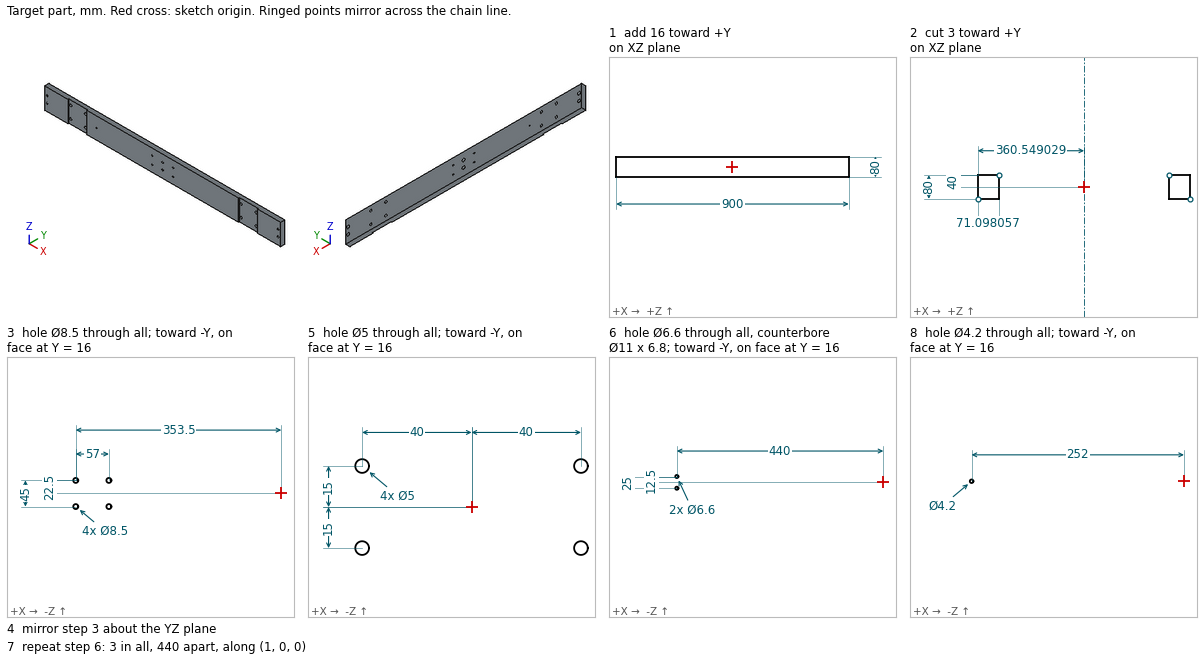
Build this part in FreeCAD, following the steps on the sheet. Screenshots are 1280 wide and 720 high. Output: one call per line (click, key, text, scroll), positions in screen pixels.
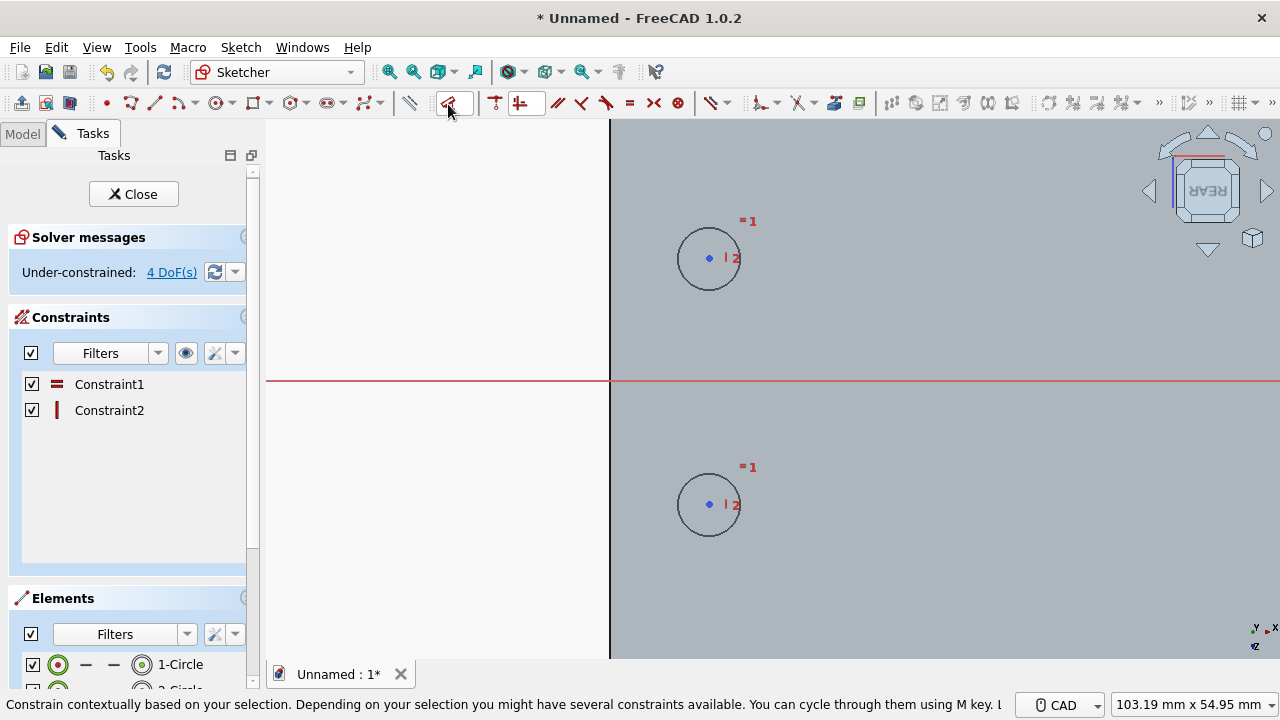
click(731, 237)
click(754, 214)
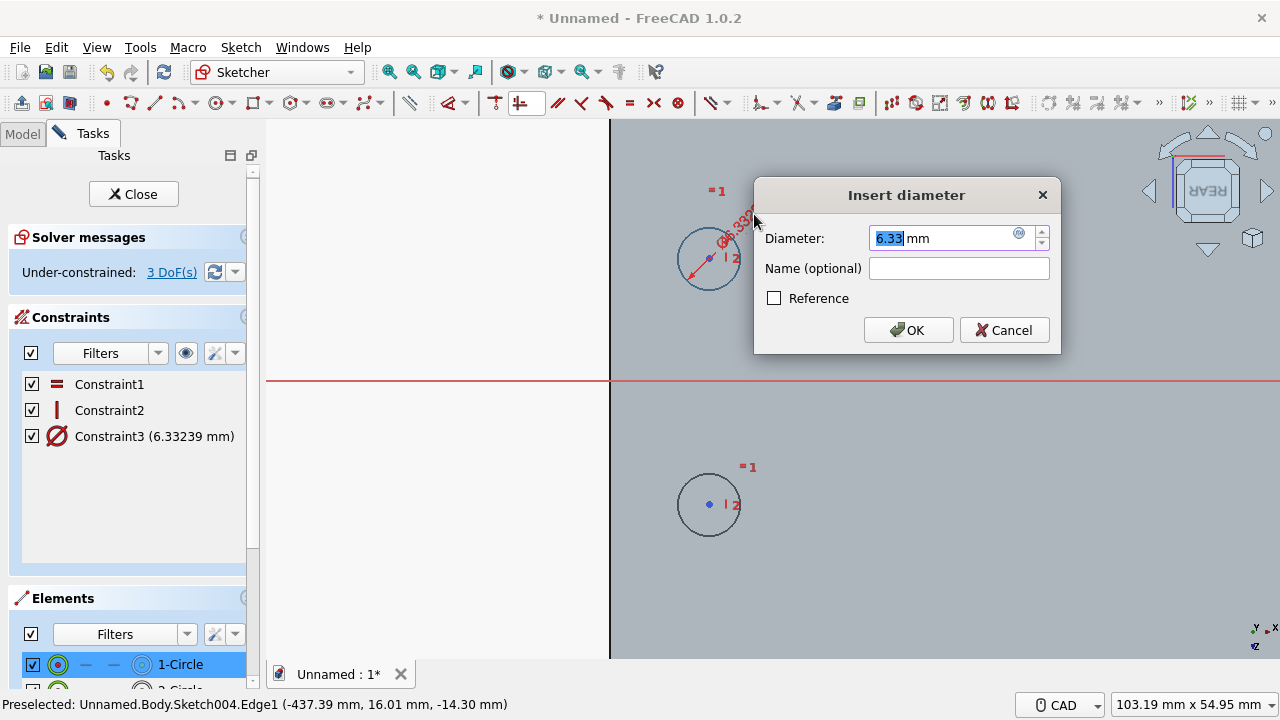
text(6.6)
key(Return)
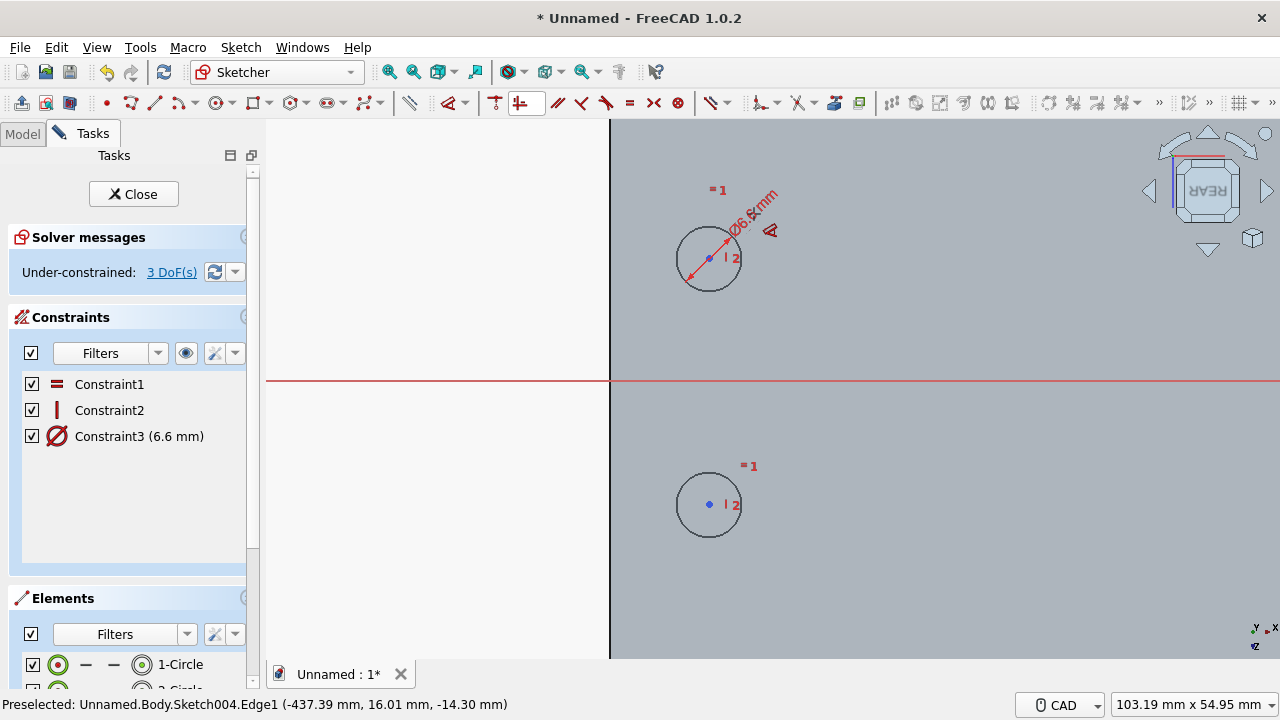
click(709, 259)
click(912, 225)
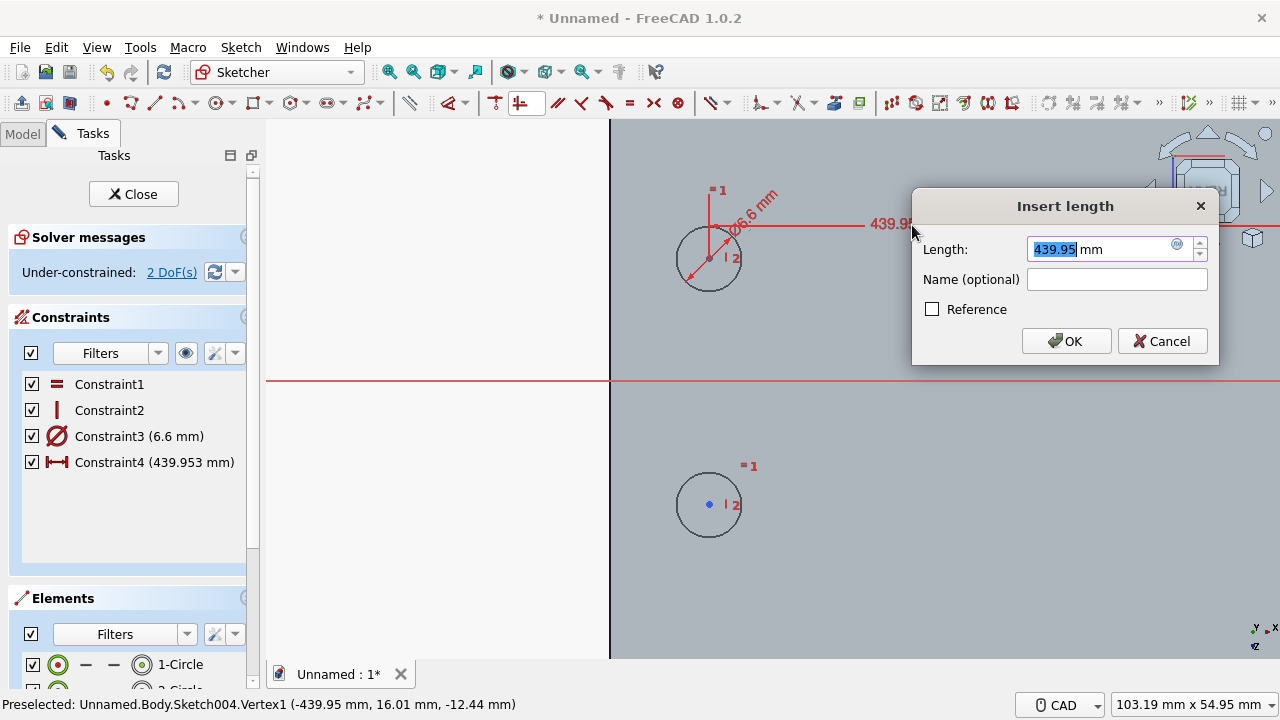
text(440)
key(Return)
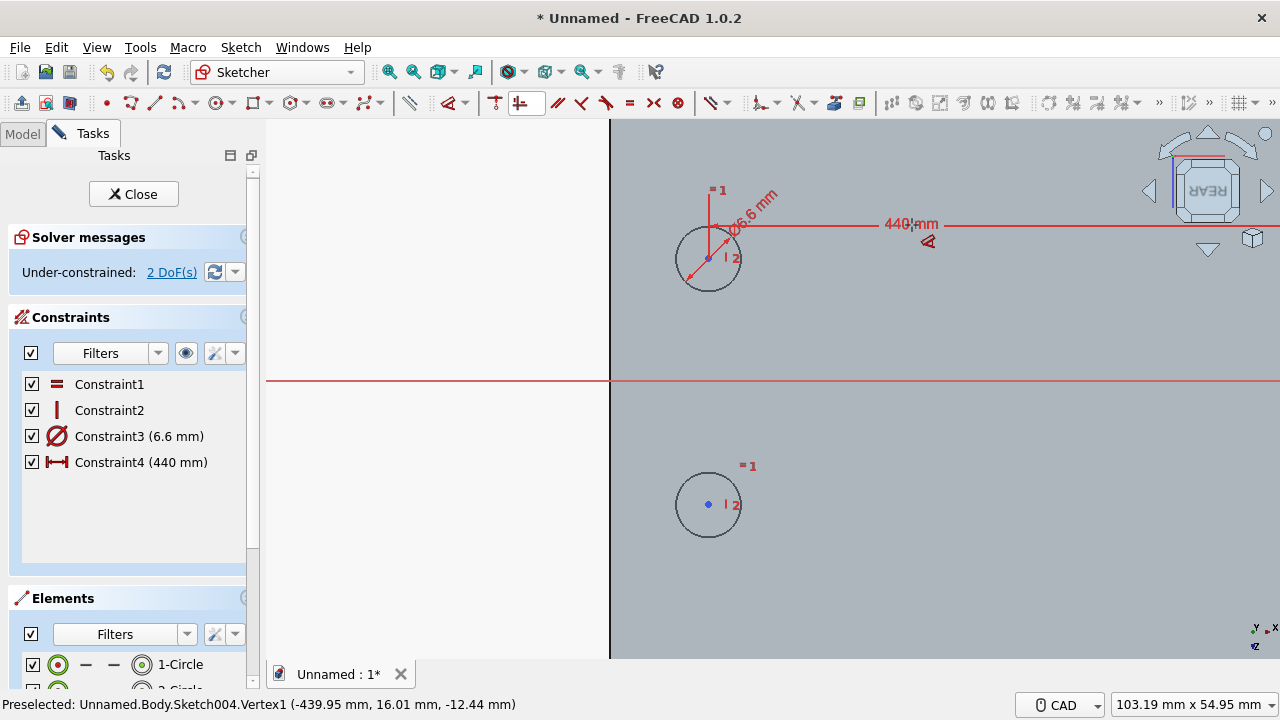
click(709, 259)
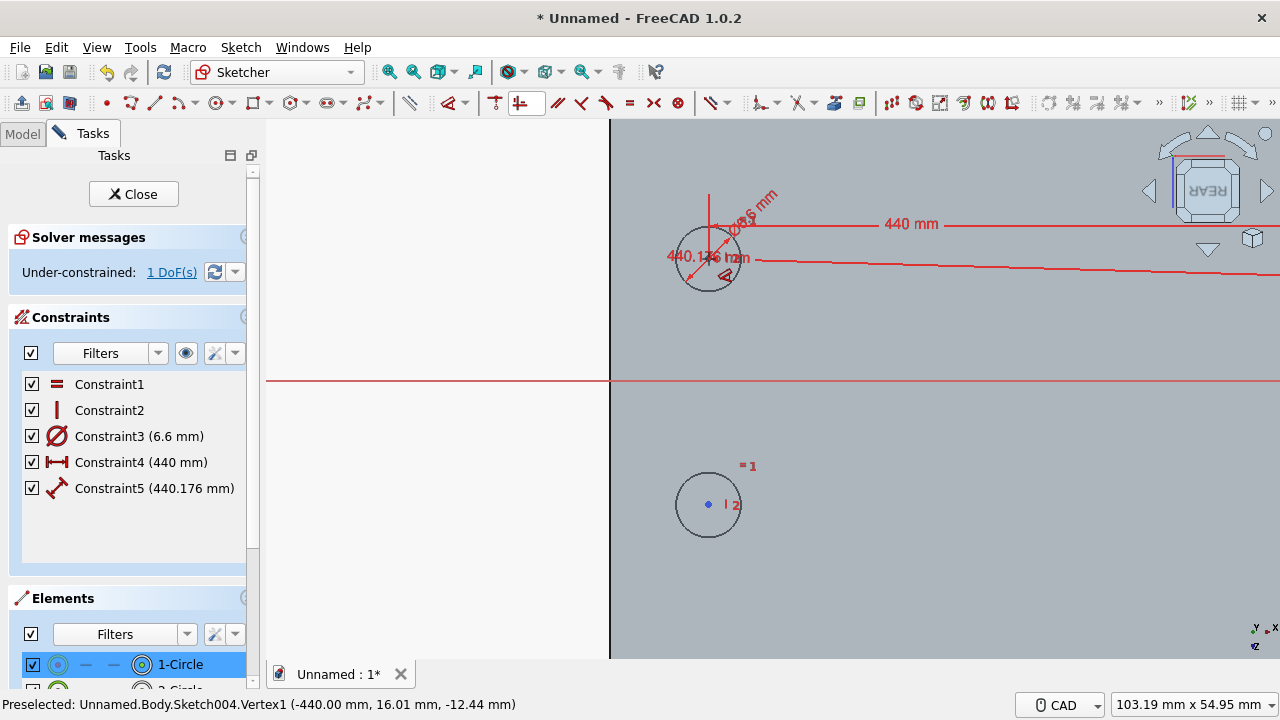
click(709, 505)
click(743, 325)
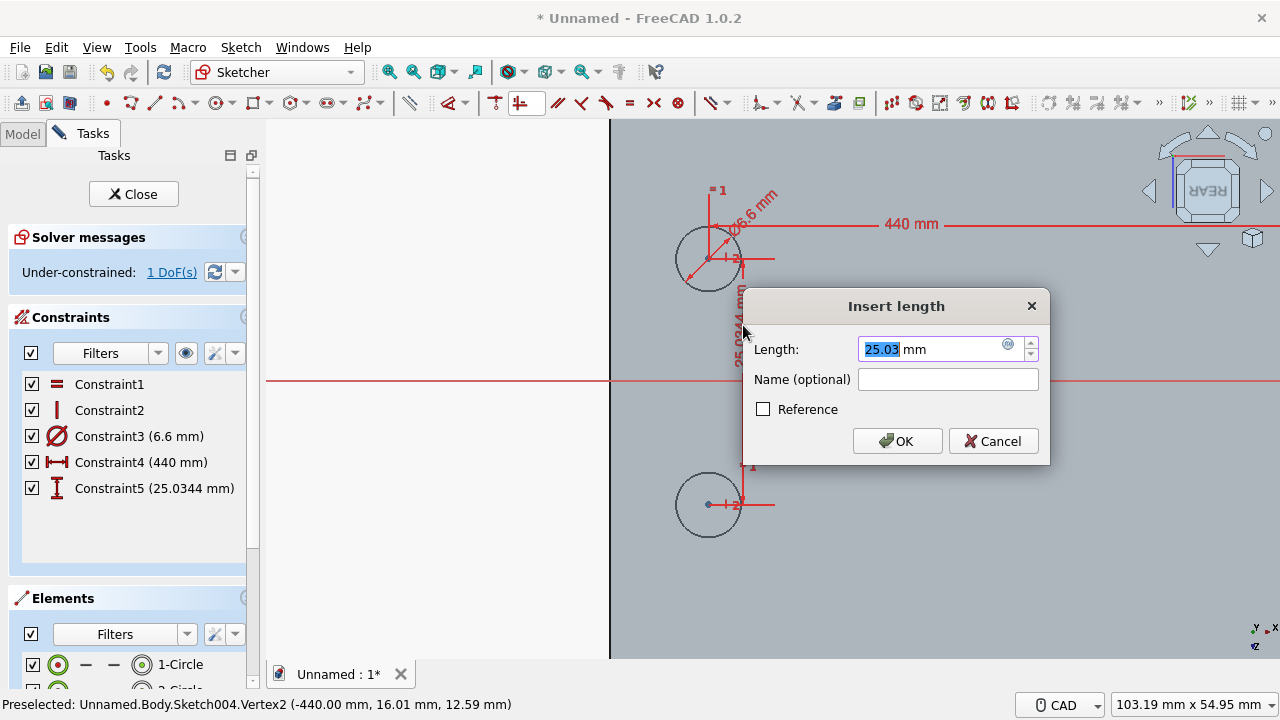
text(25)
key(Return)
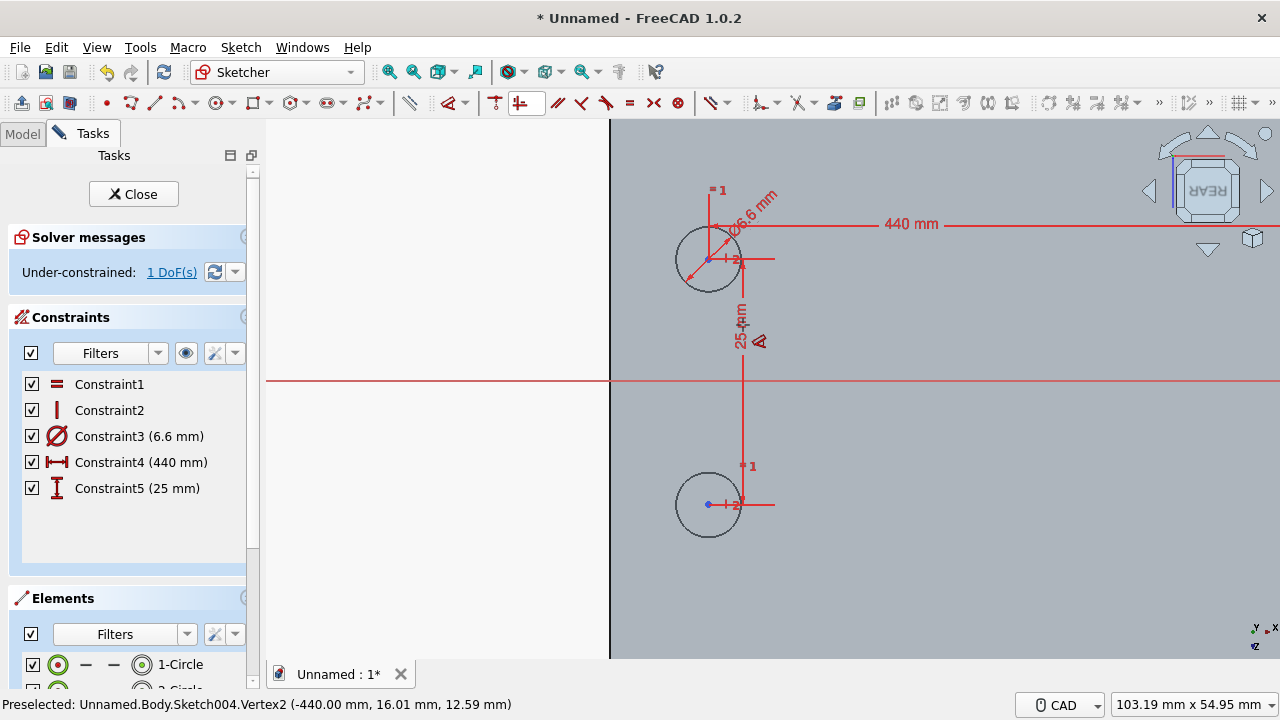
click(709, 259)
click(675, 292)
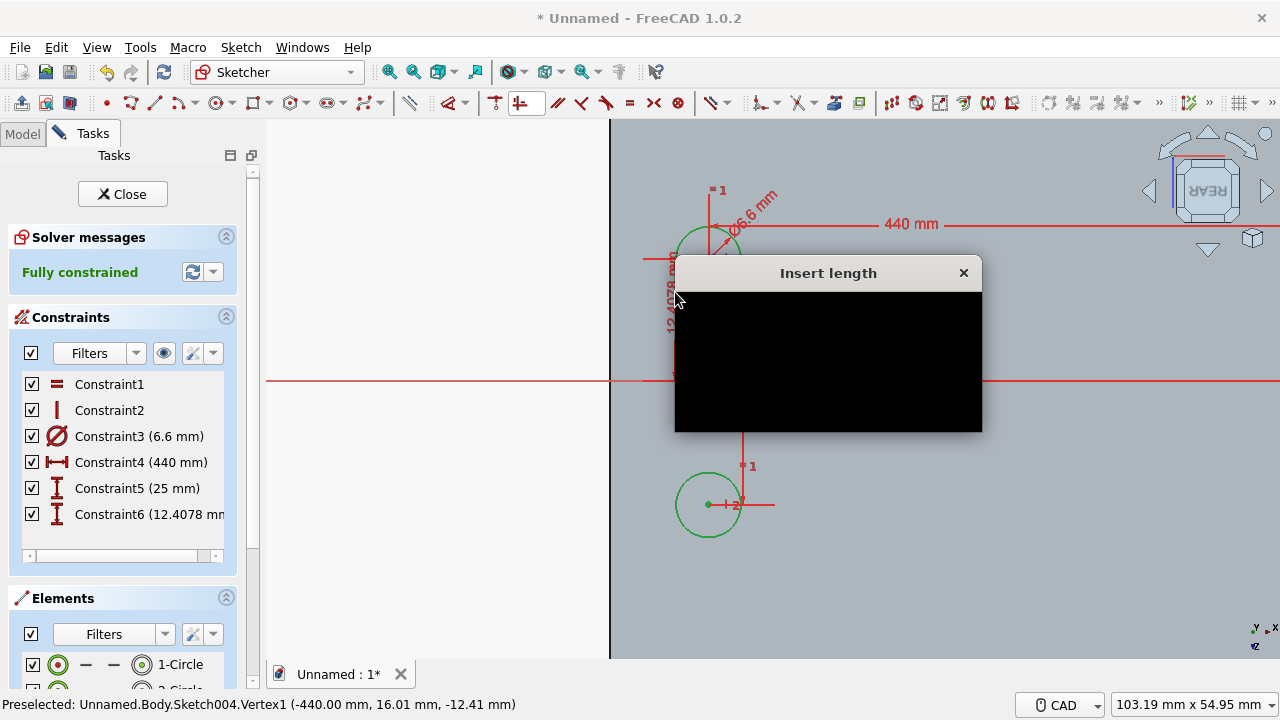
text(12.5)
key(Return)
key(Escape)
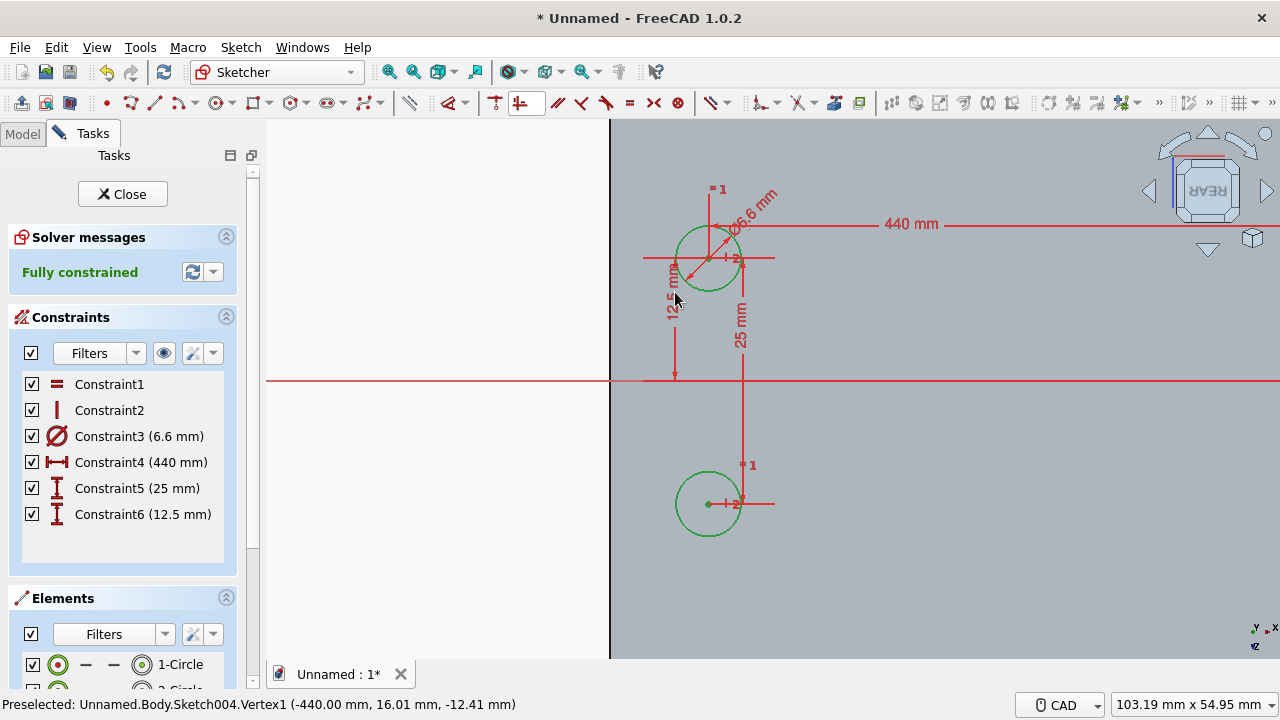
click(123, 194)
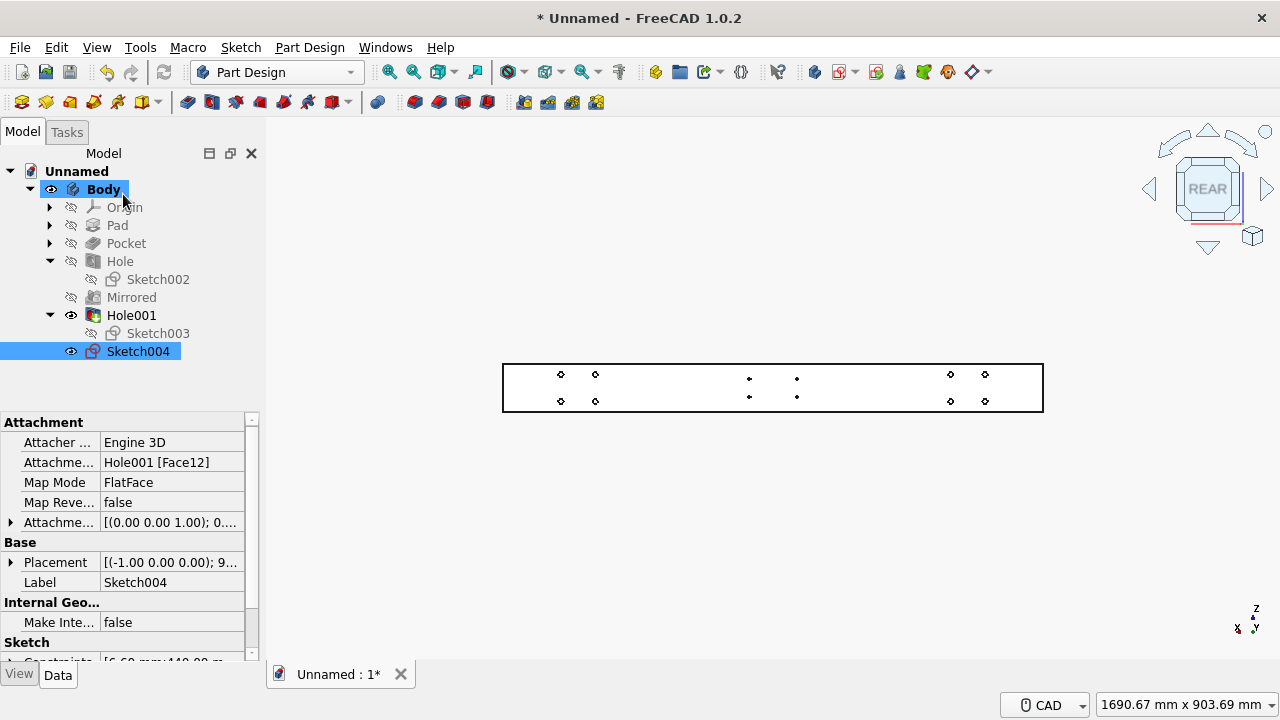
click(212, 102)